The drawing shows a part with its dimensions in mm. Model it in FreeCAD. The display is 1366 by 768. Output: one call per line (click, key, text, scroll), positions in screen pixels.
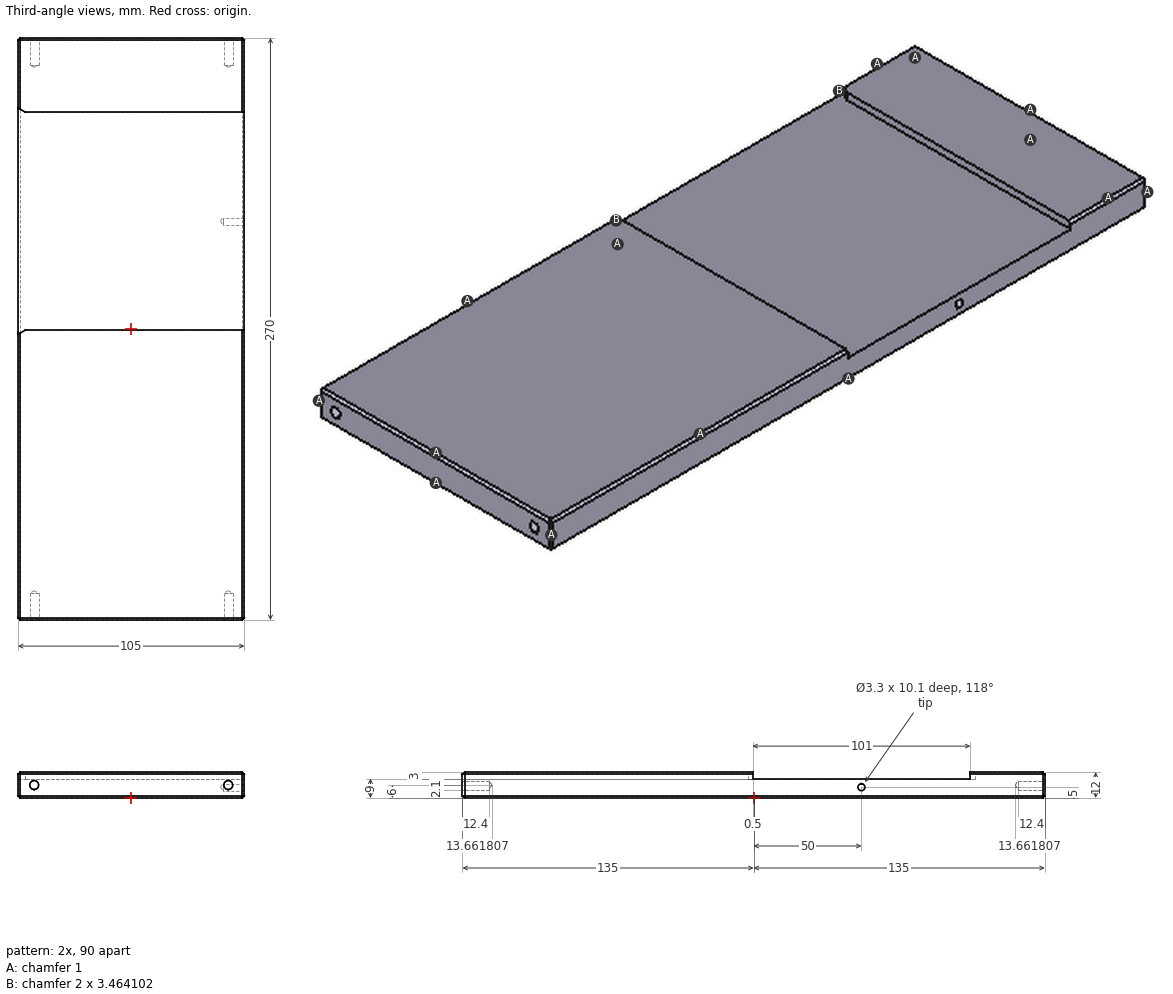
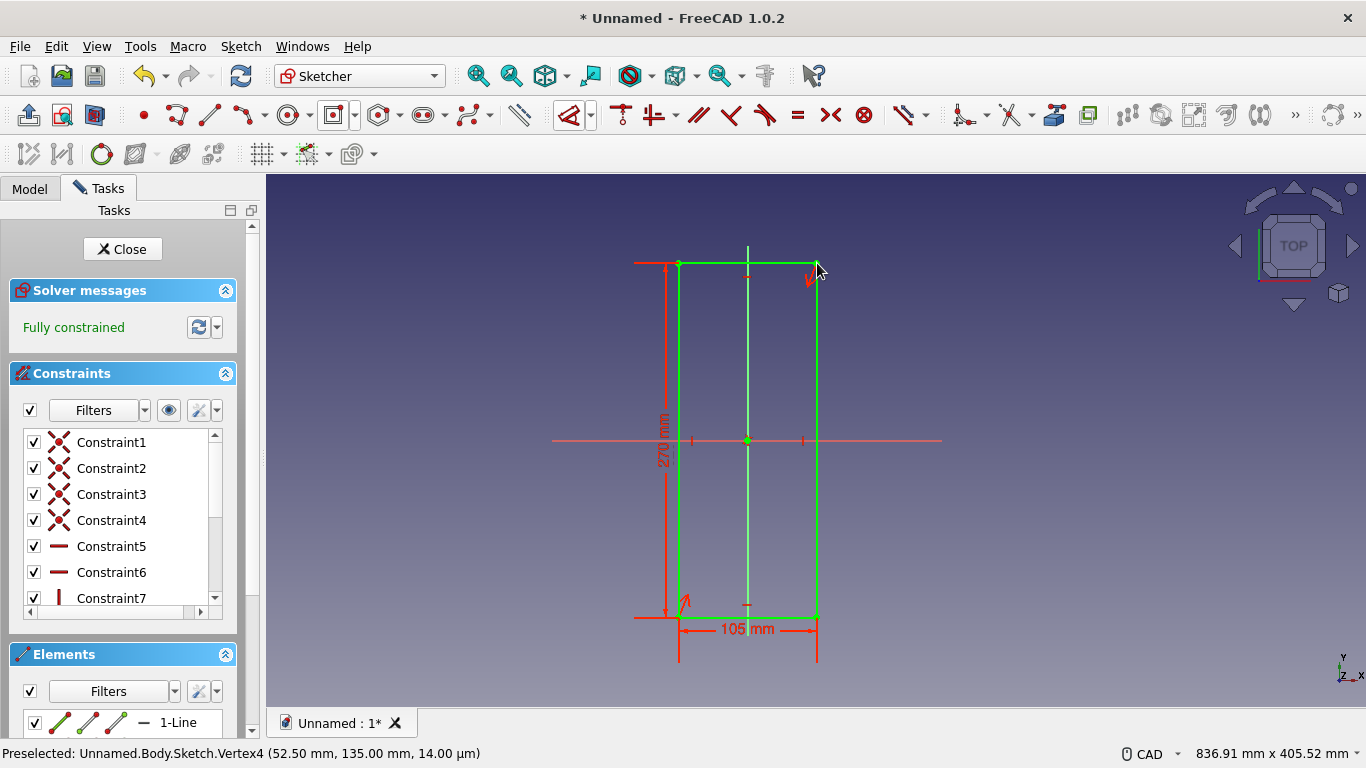
click(123, 249)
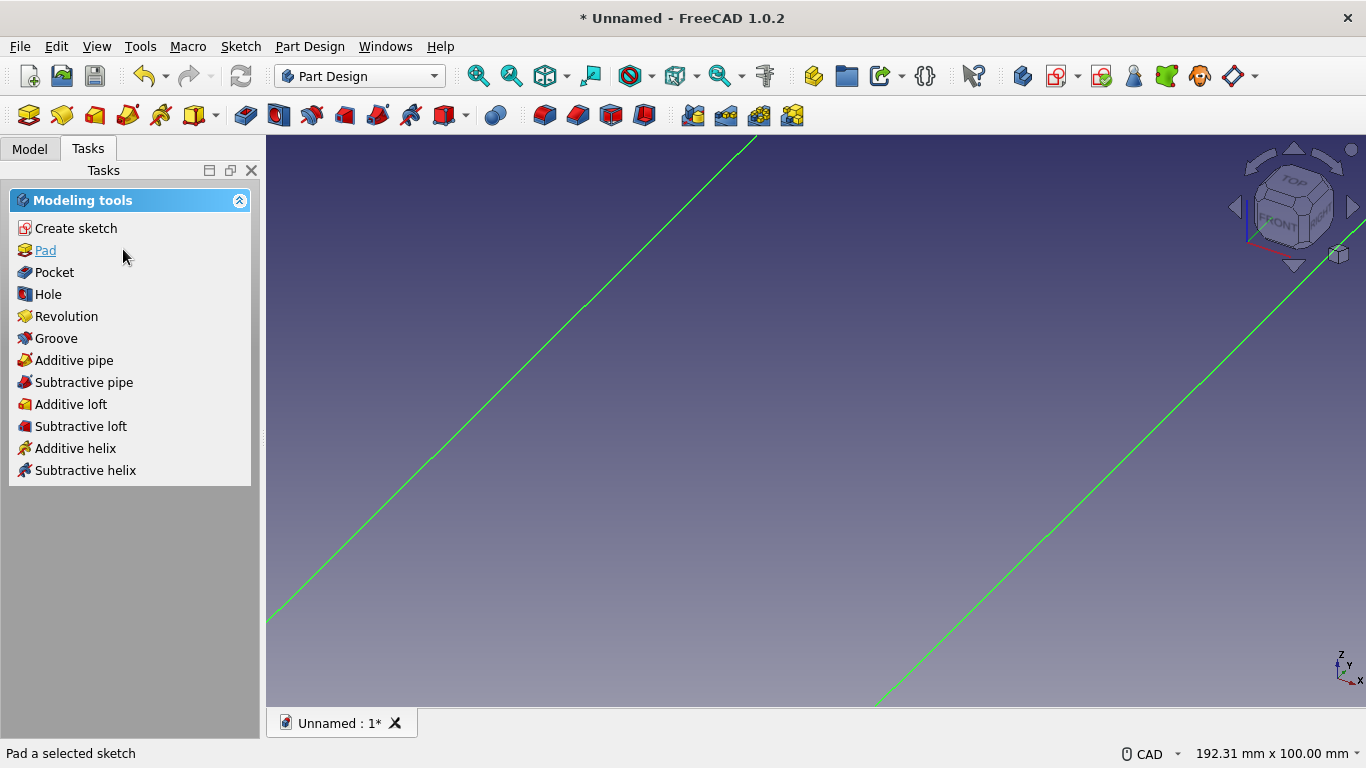
click(29, 116)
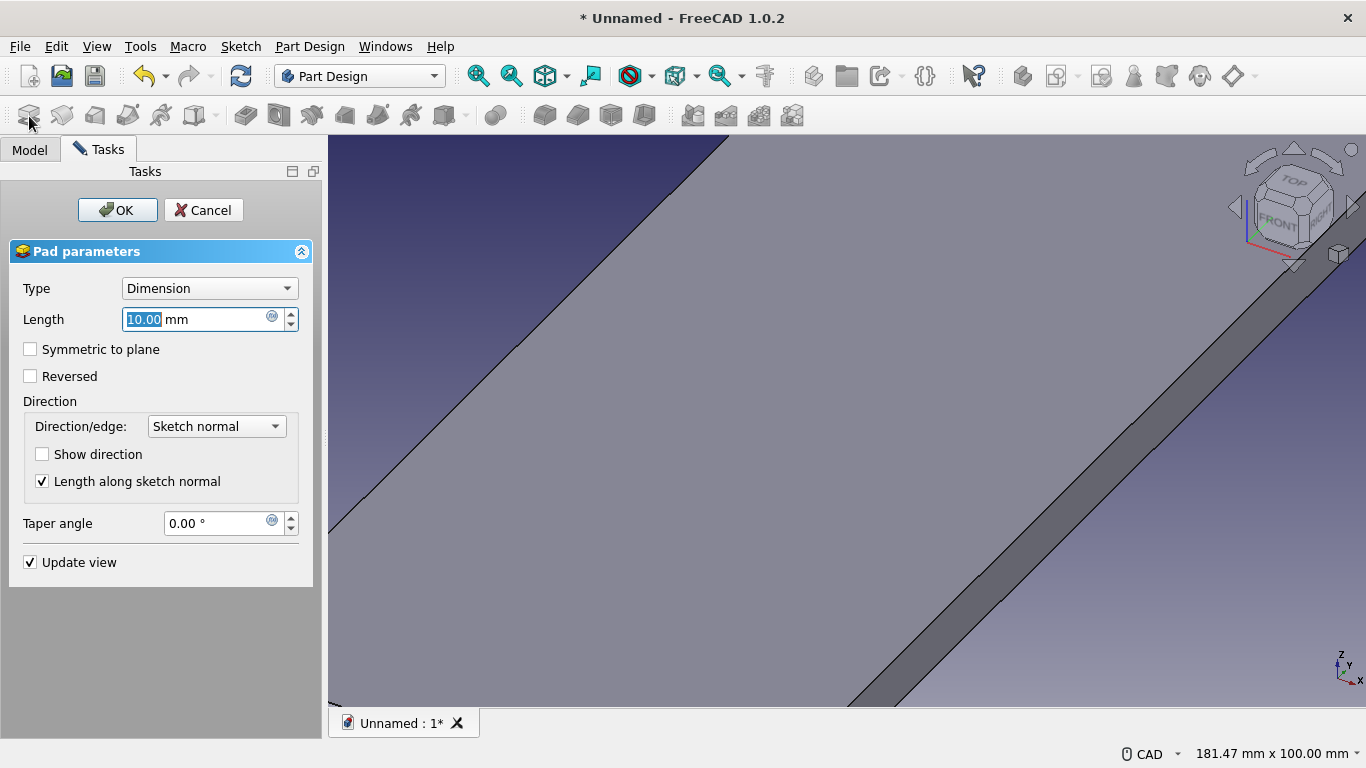
text(12)
key(Tab)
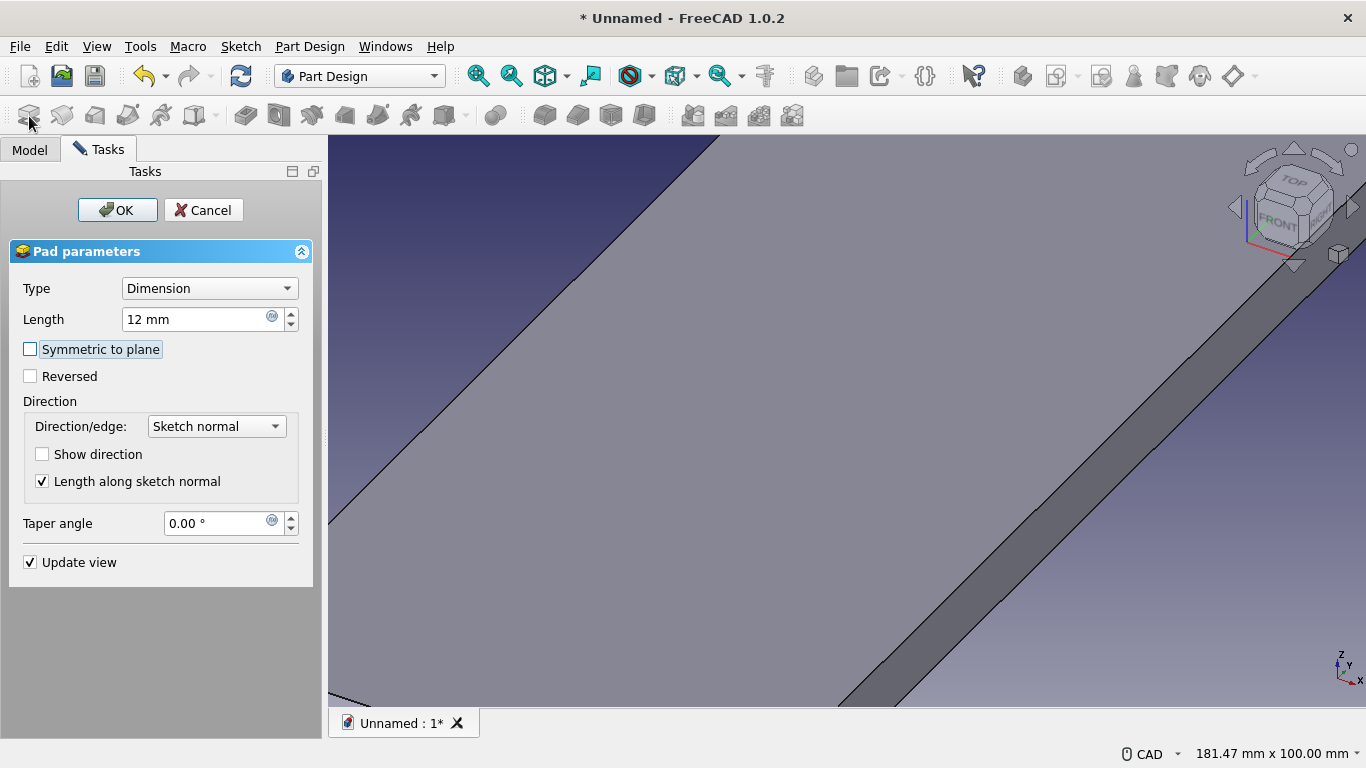
click(118, 210)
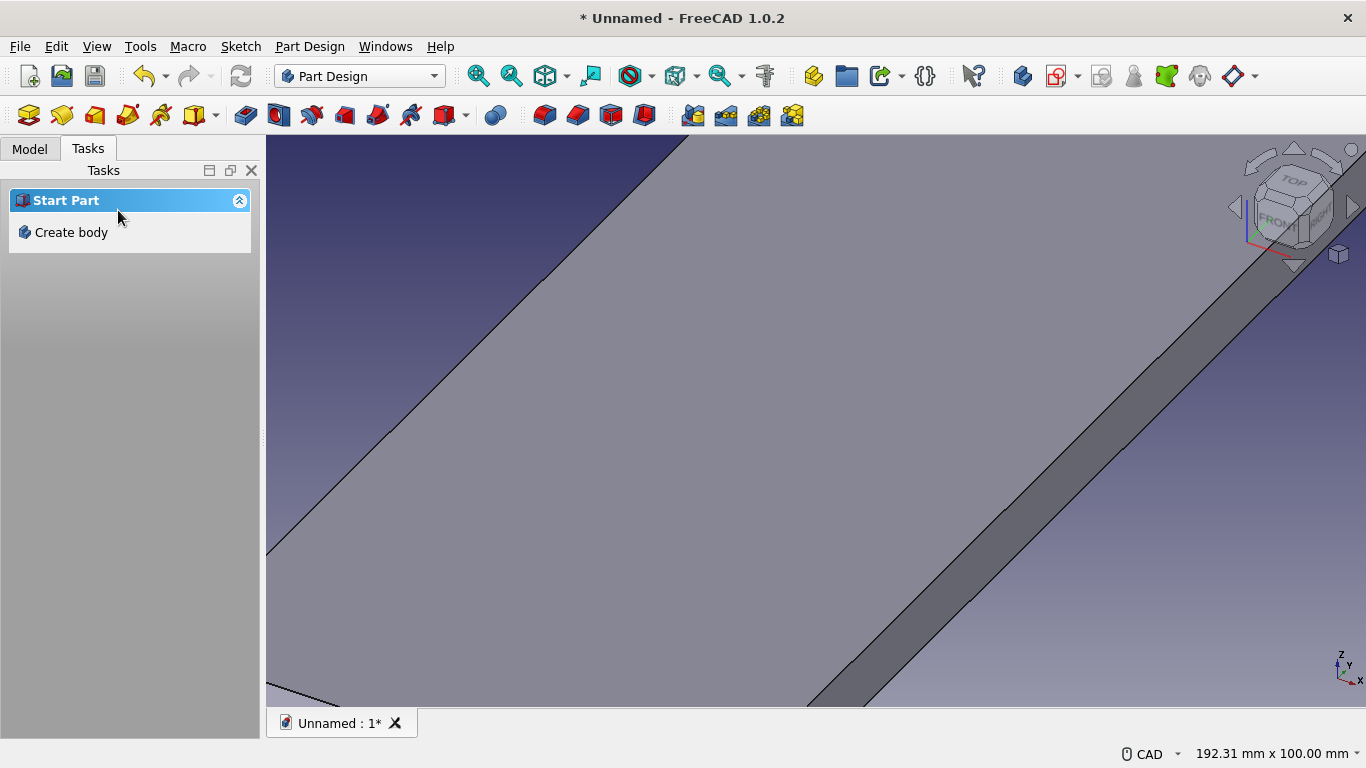
click(479, 76)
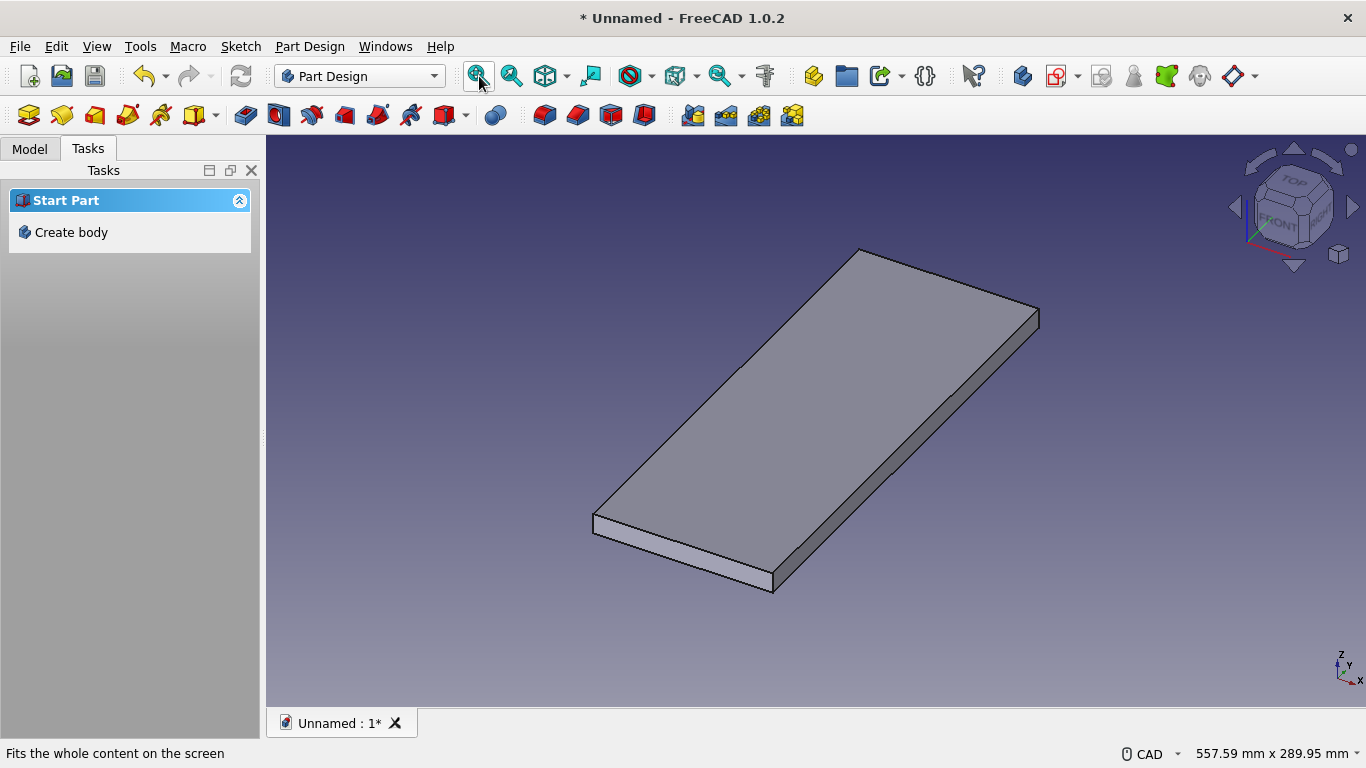
key(0)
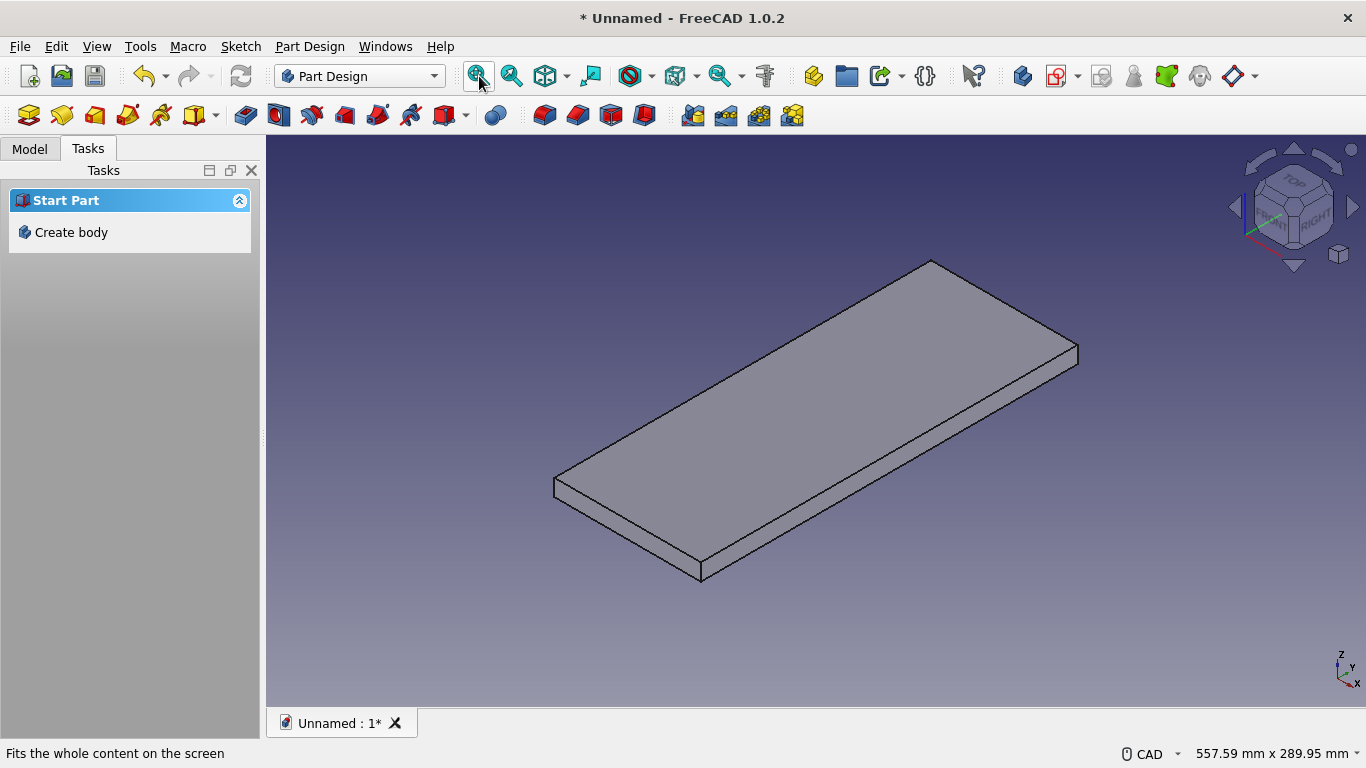
key(3)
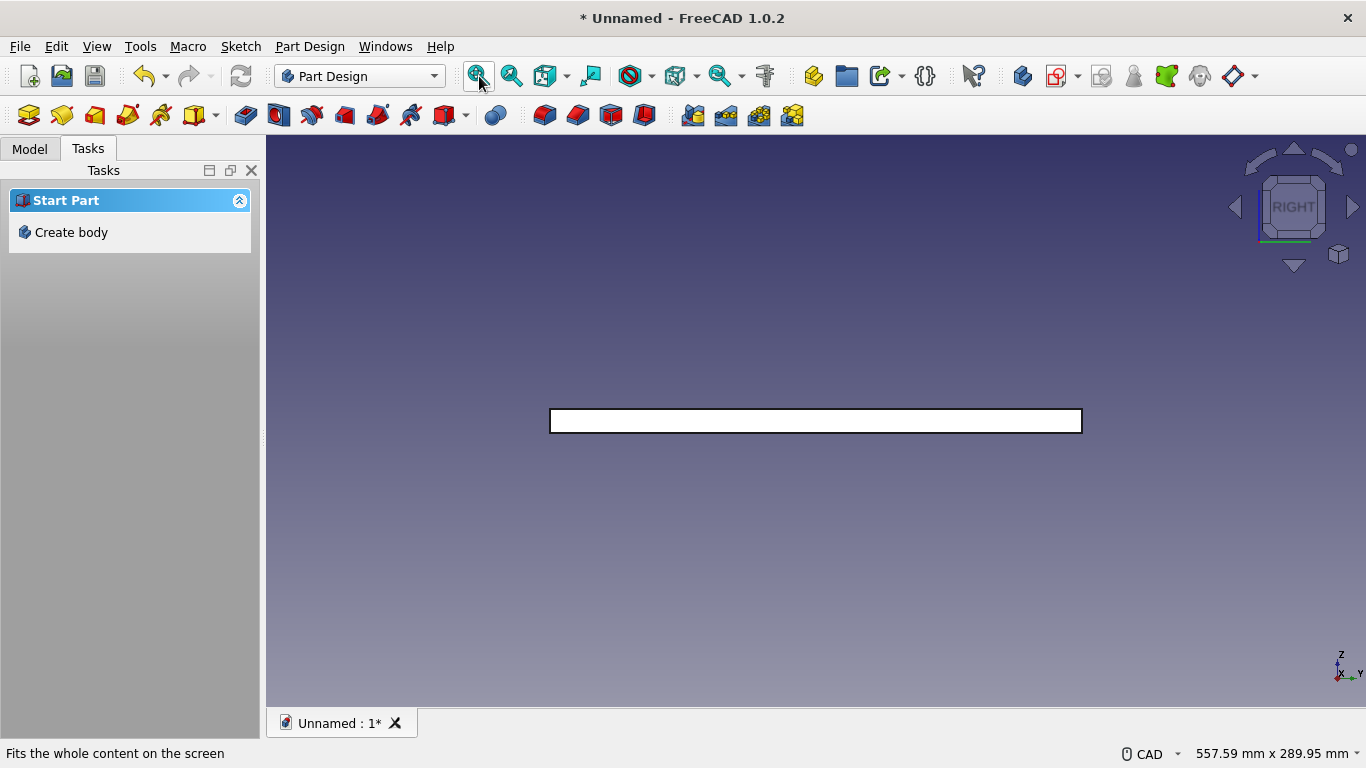
click(1044, 420)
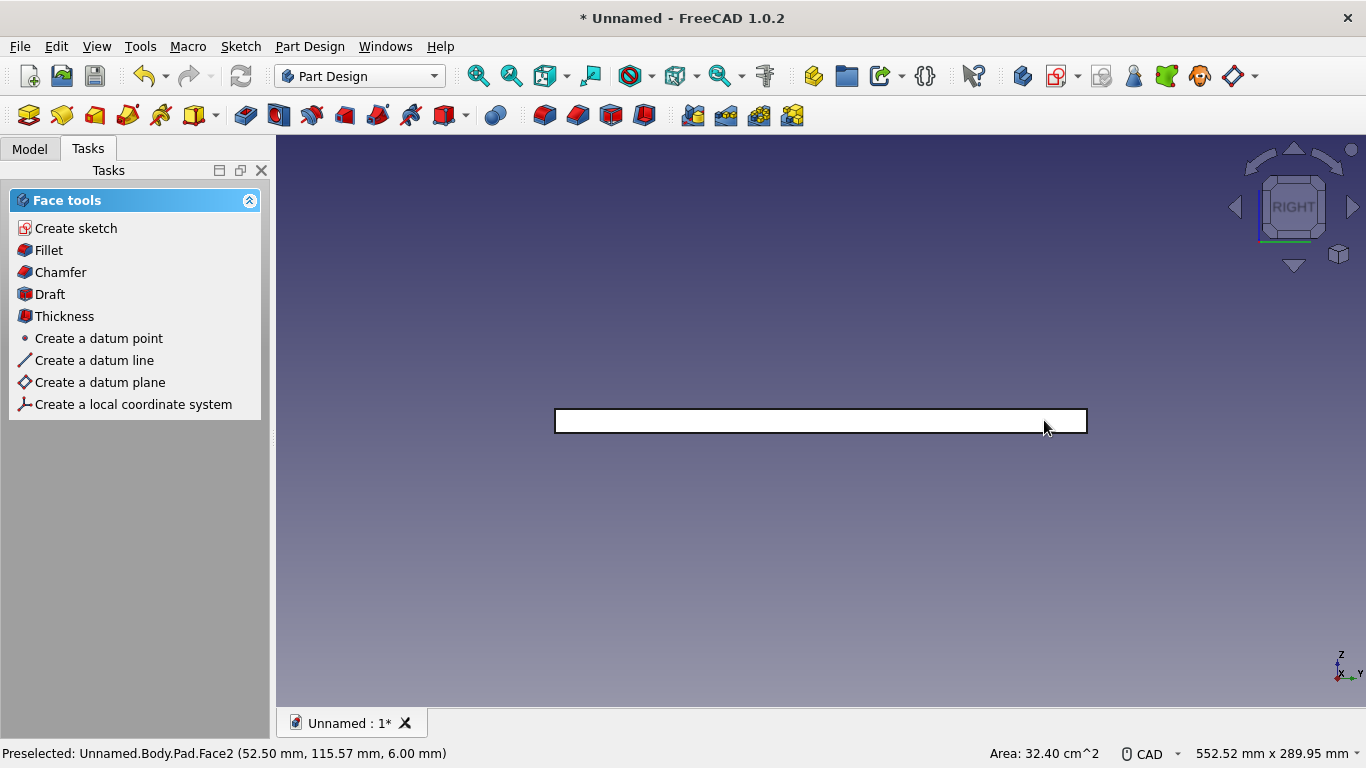
click(1056, 76)